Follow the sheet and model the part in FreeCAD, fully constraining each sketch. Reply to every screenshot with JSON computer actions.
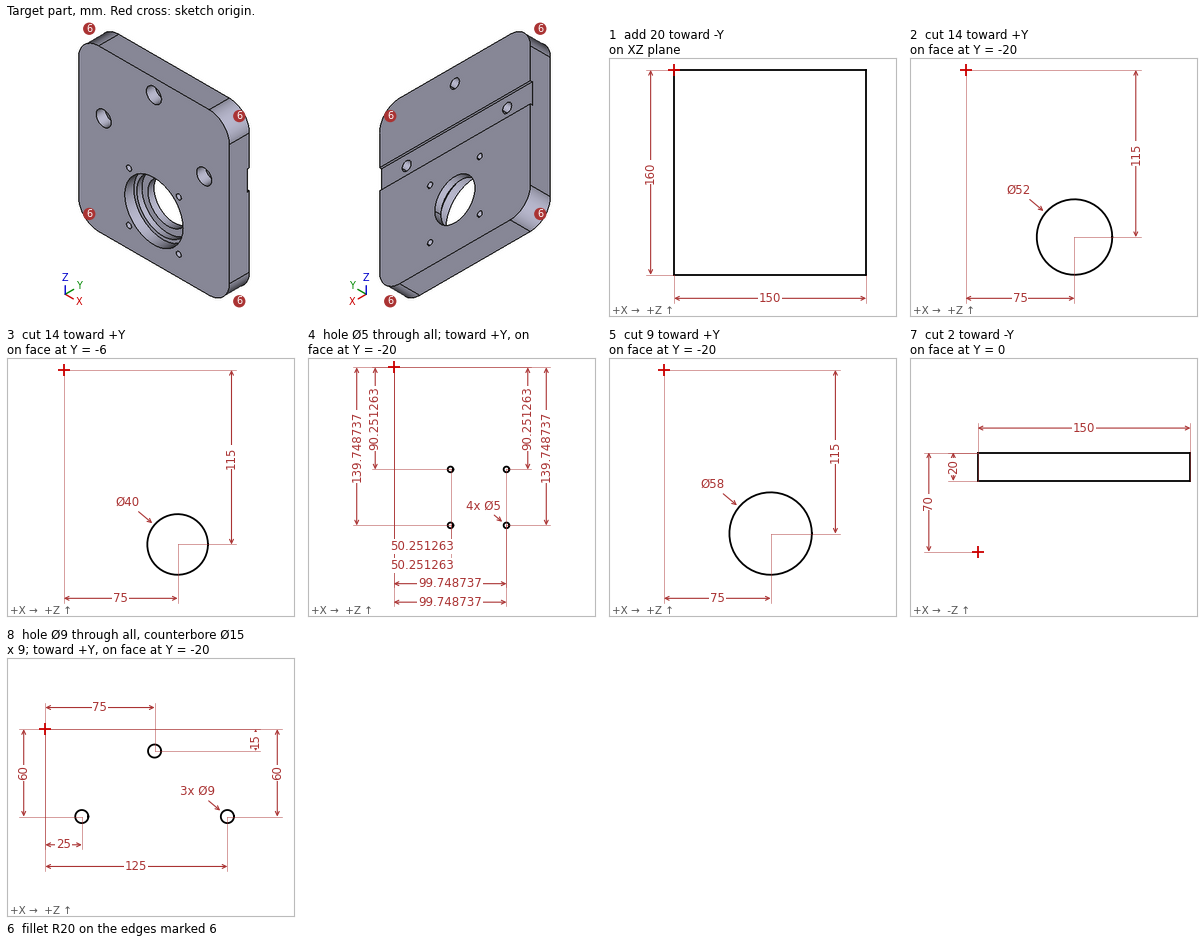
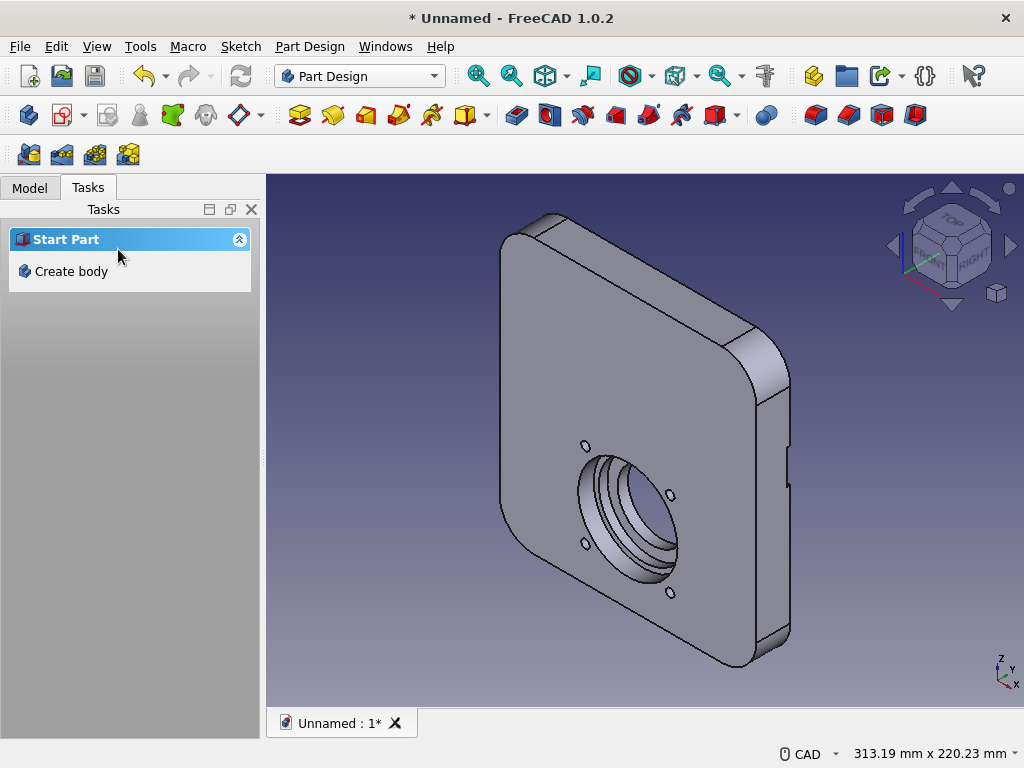
{"action": "left_click", "coordinate": [665, 380]}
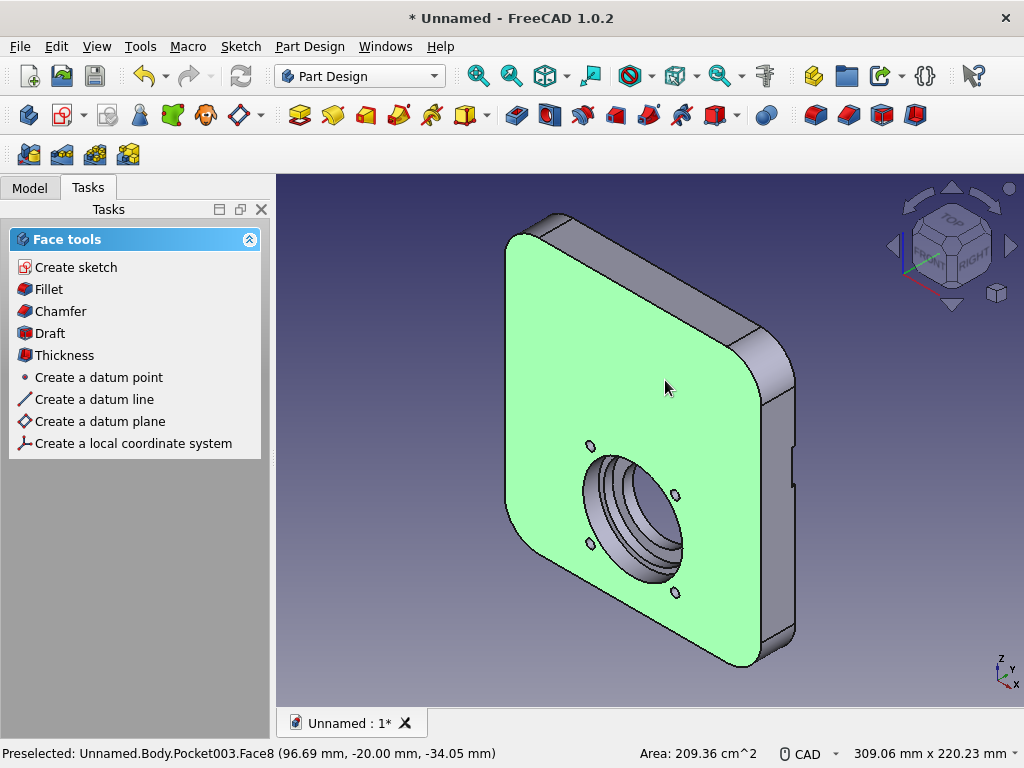
{"action": "left_click", "coordinate": [62, 116]}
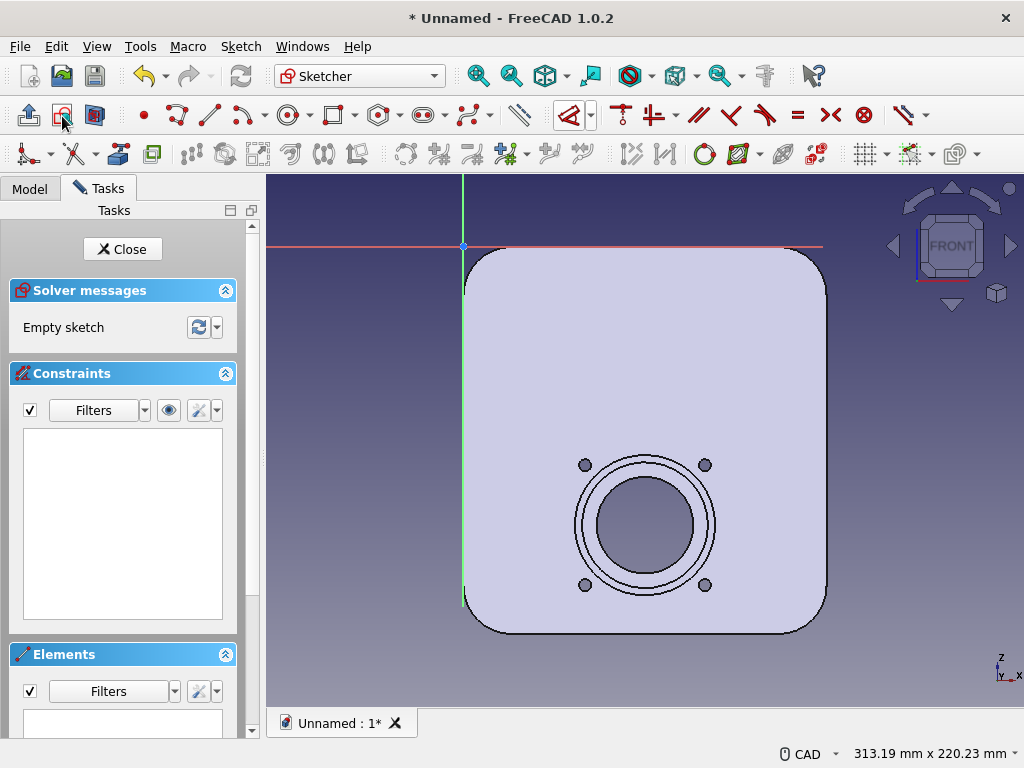
{"action": "left_click", "coordinate": [288, 116]}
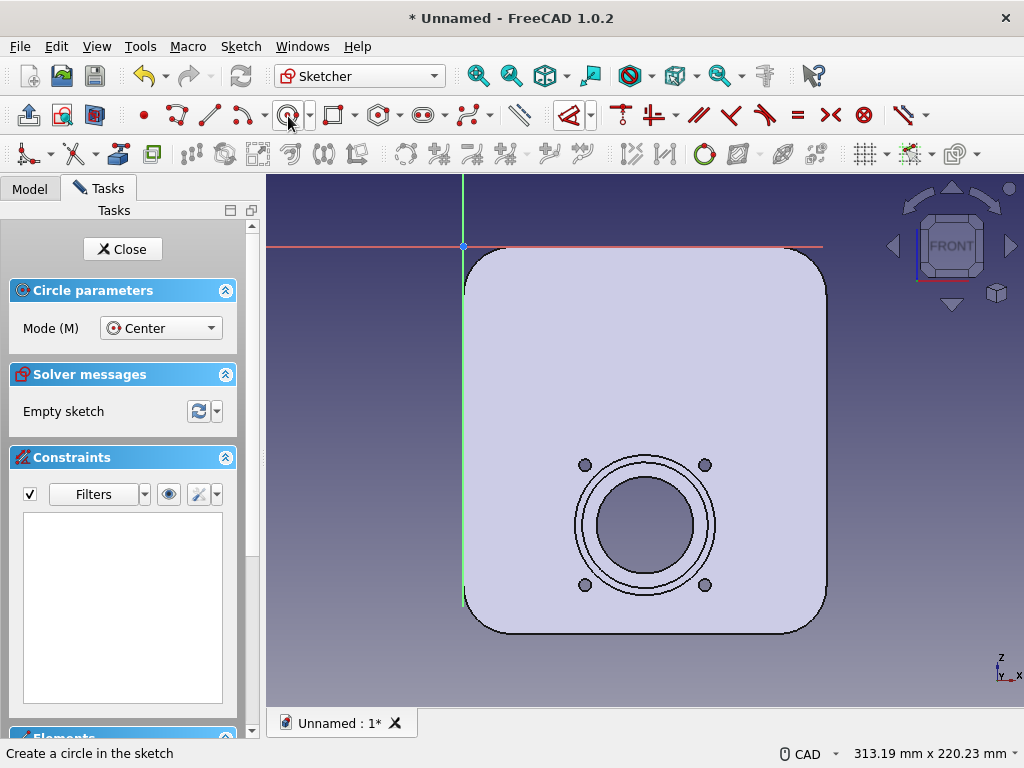
{"action": "scroll", "coordinate": [766, 392], "scroll_direction": "up", "scroll_amount": 4}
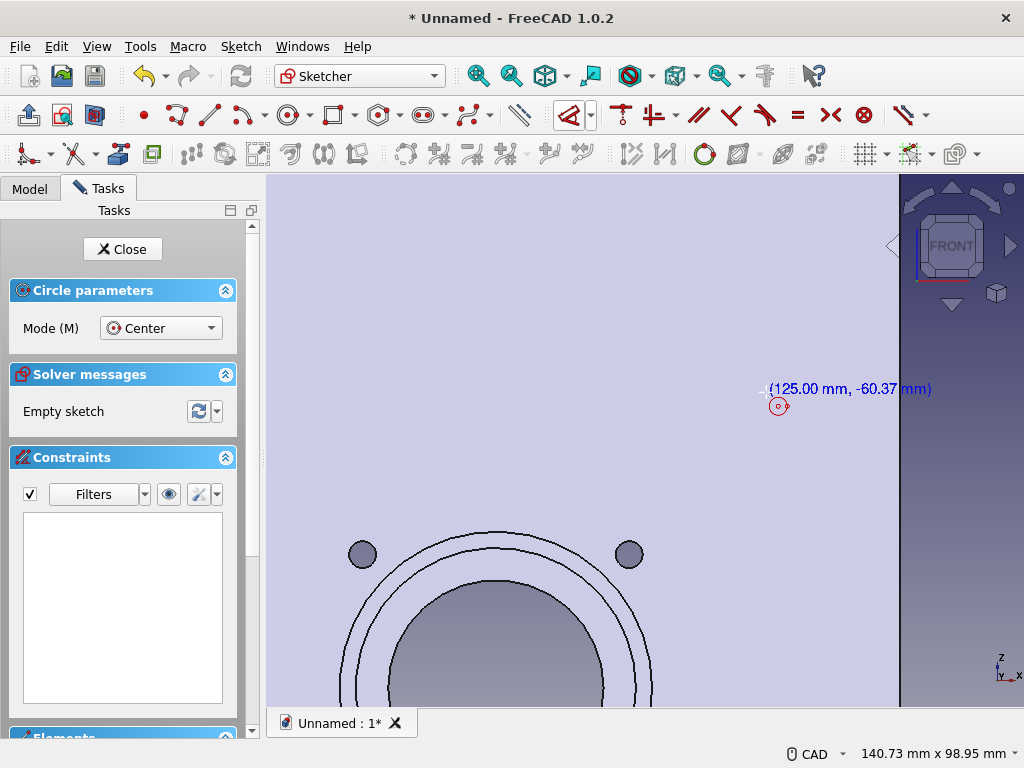
{"action": "left_click", "coordinate": [765, 392]}
{"action": "left_click", "coordinate": [782, 375]}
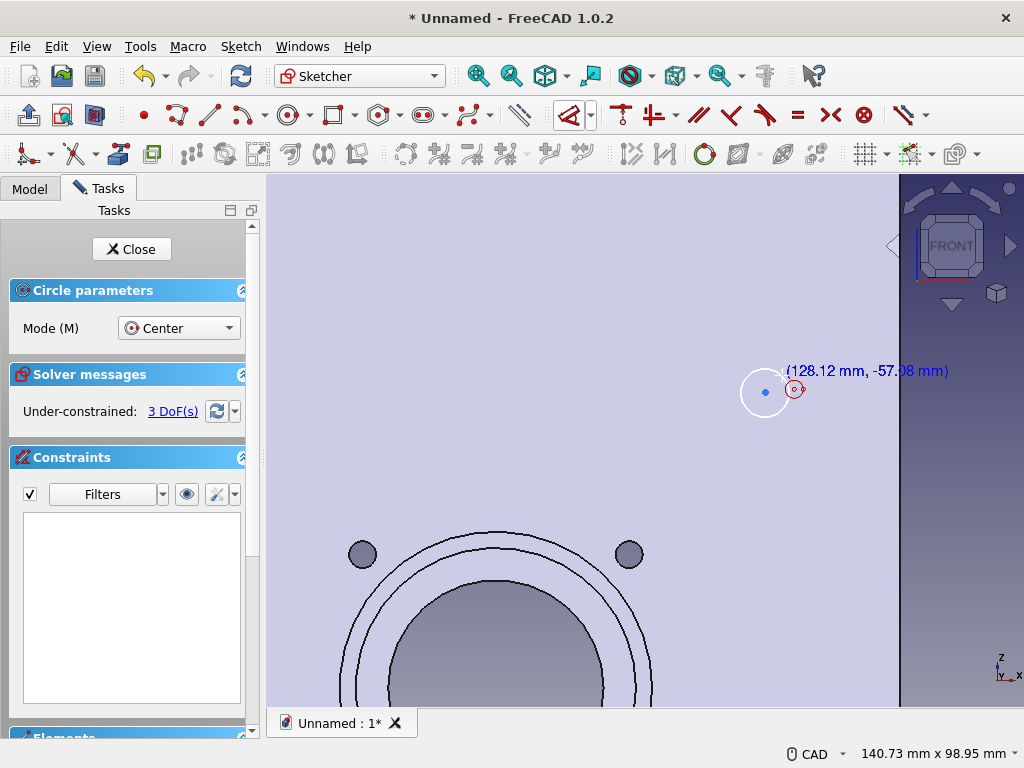
{"action": "scroll", "coordinate": [742, 679], "scroll_direction": "down", "scroll_amount": 3}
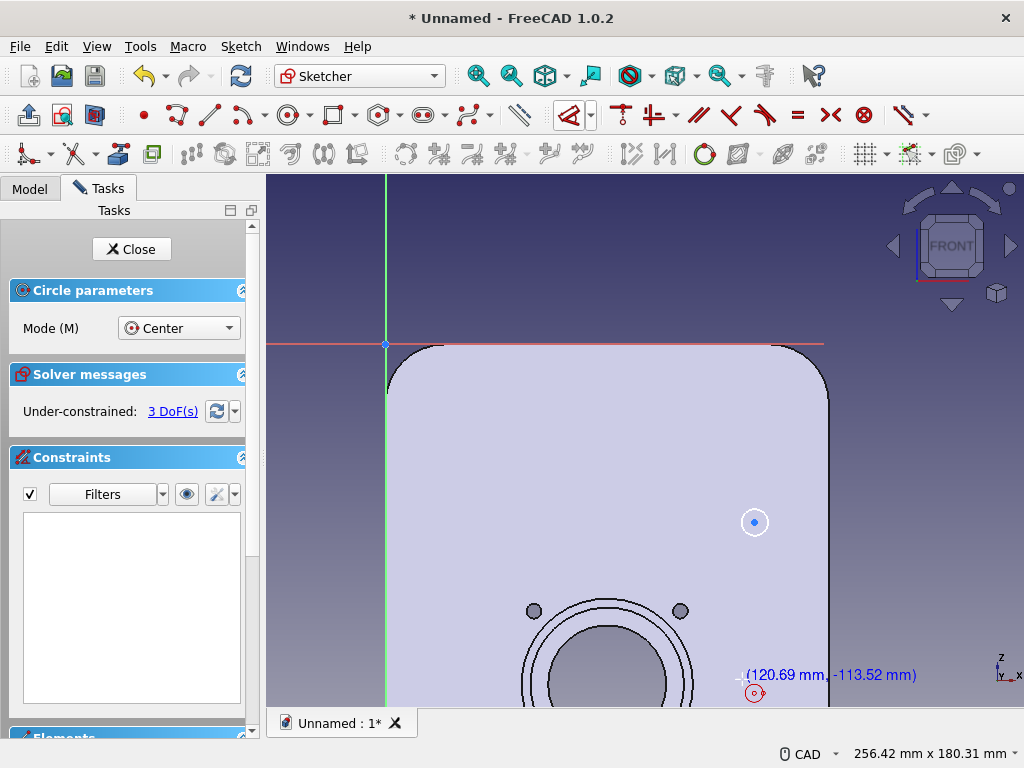
{"action": "scroll", "coordinate": [459, 522], "scroll_direction": "up", "scroll_amount": 3}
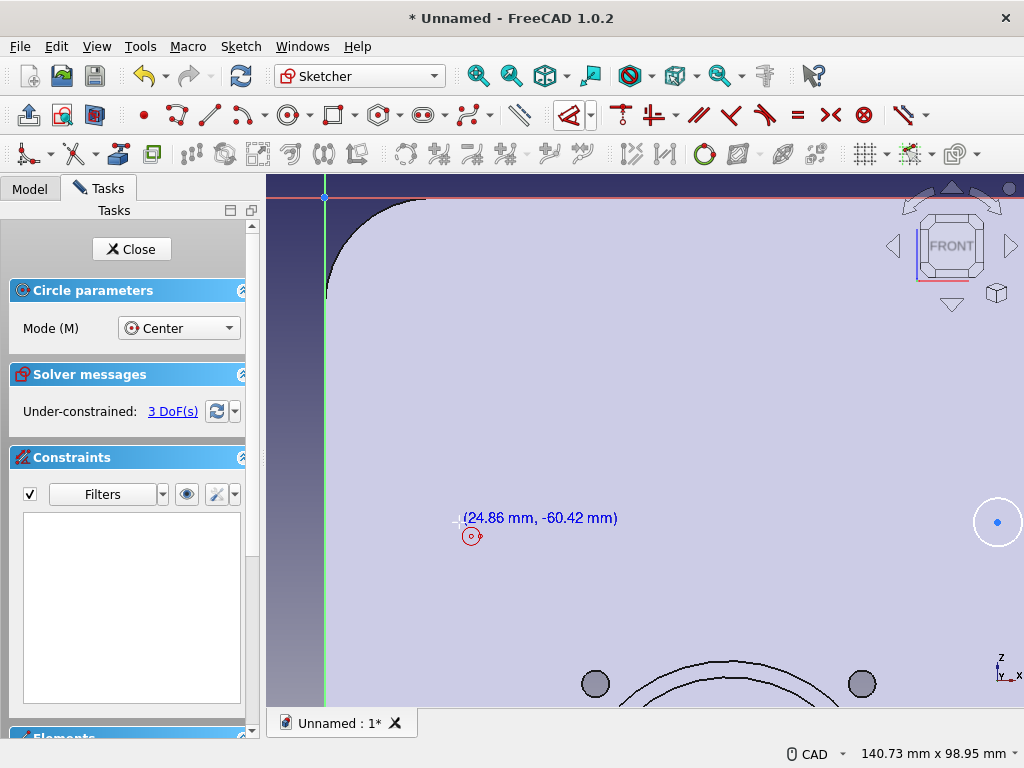
{"action": "left_click", "coordinate": [460, 521]}
{"action": "left_click", "coordinate": [477, 504]}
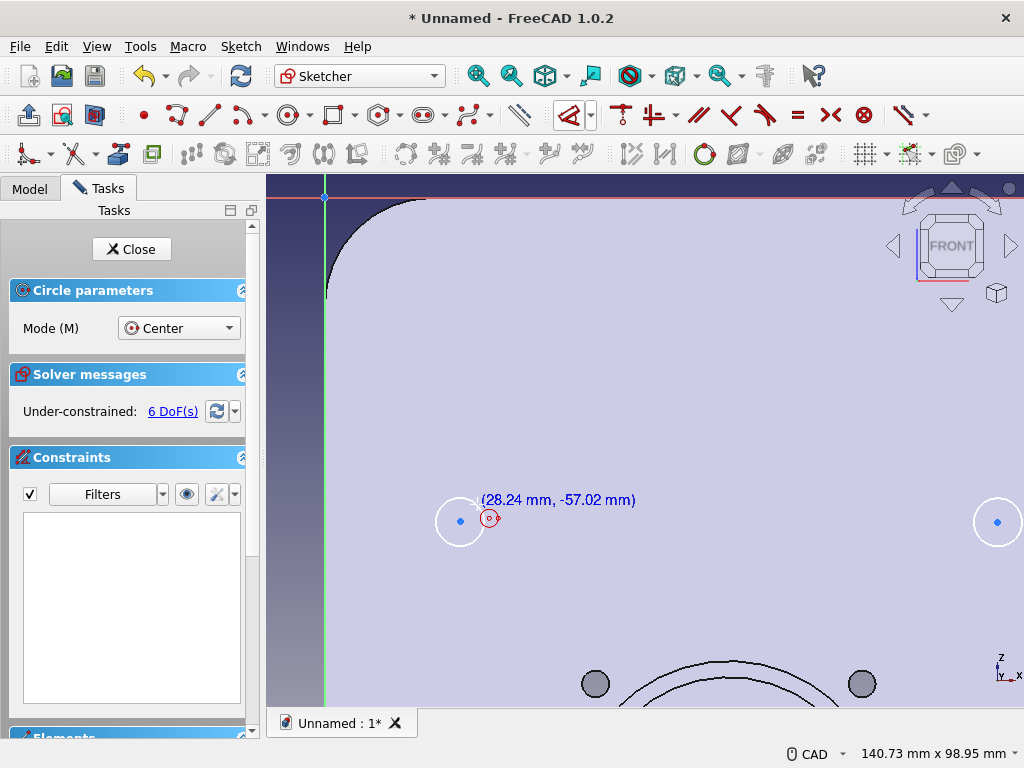
{"action": "left_click", "coordinate": [729, 279]}
{"action": "left_click", "coordinate": [746, 262]}
{"action": "key", "text": "Escape"}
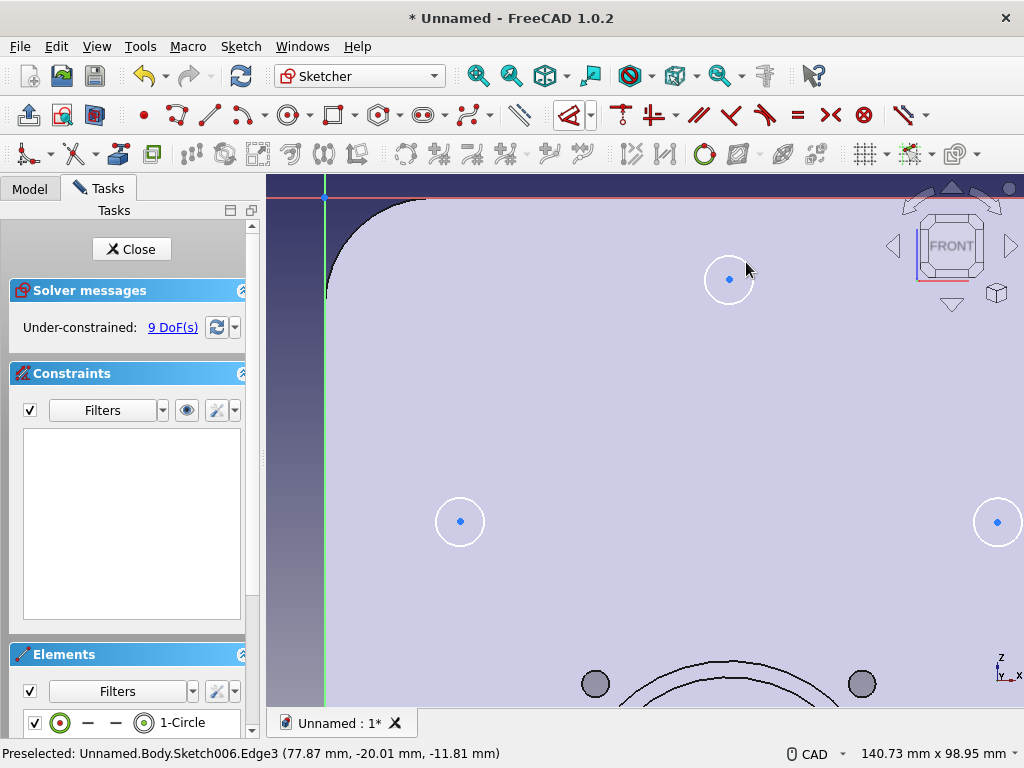
{"action": "scroll", "coordinate": [458, 524], "scroll_direction": "down", "scroll_amount": 3}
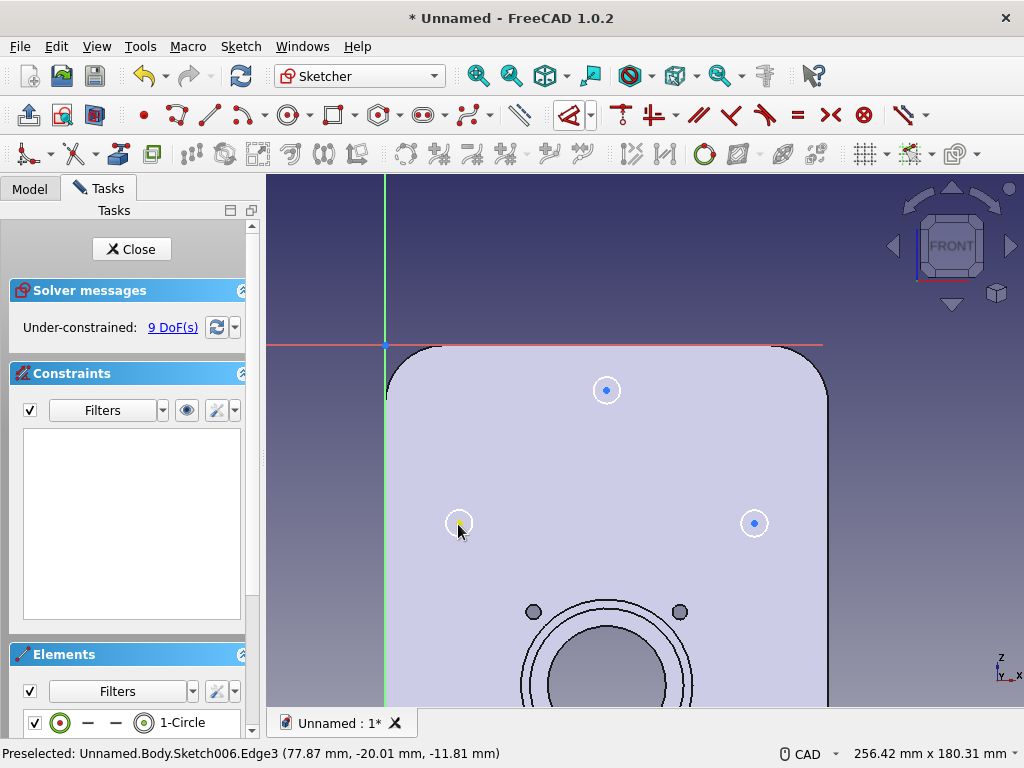
{"action": "left_click", "coordinate": [764, 514]}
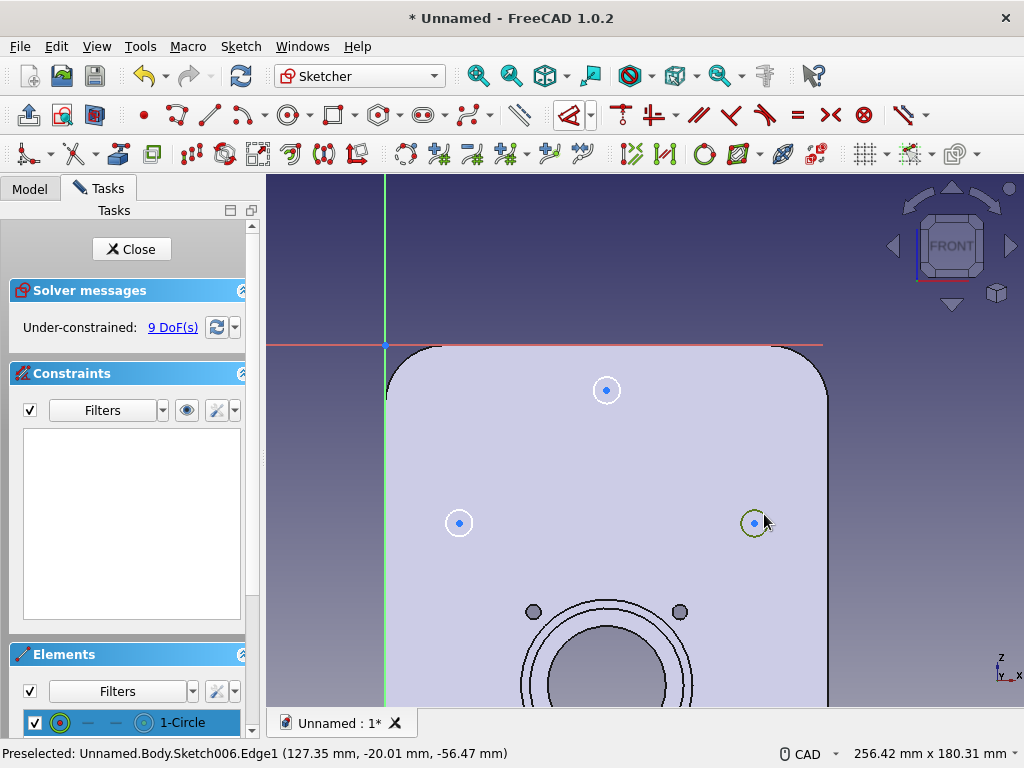
{"action": "left_click", "coordinate": [469, 514]}